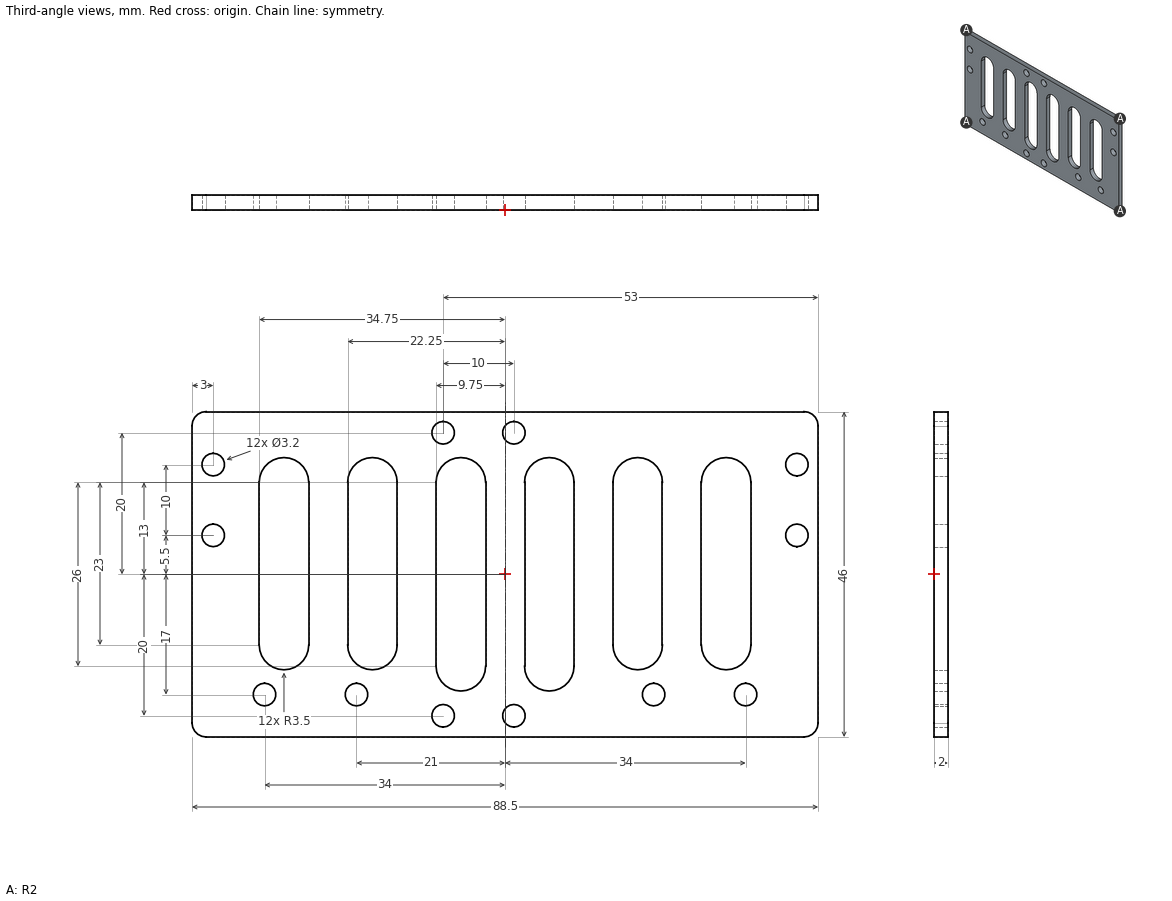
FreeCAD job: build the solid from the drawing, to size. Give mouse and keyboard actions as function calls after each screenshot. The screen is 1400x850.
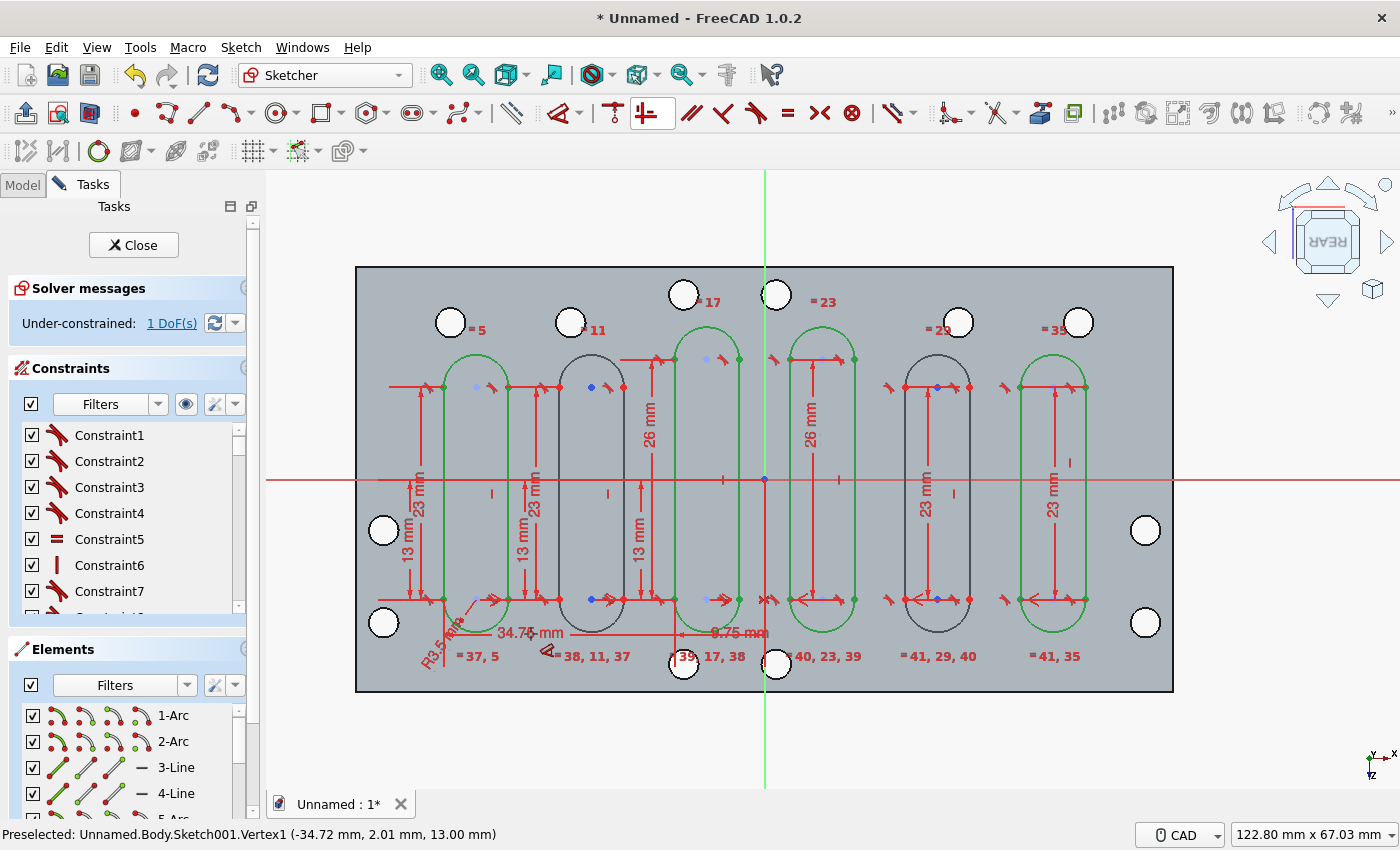
click(559, 600)
click(662, 634)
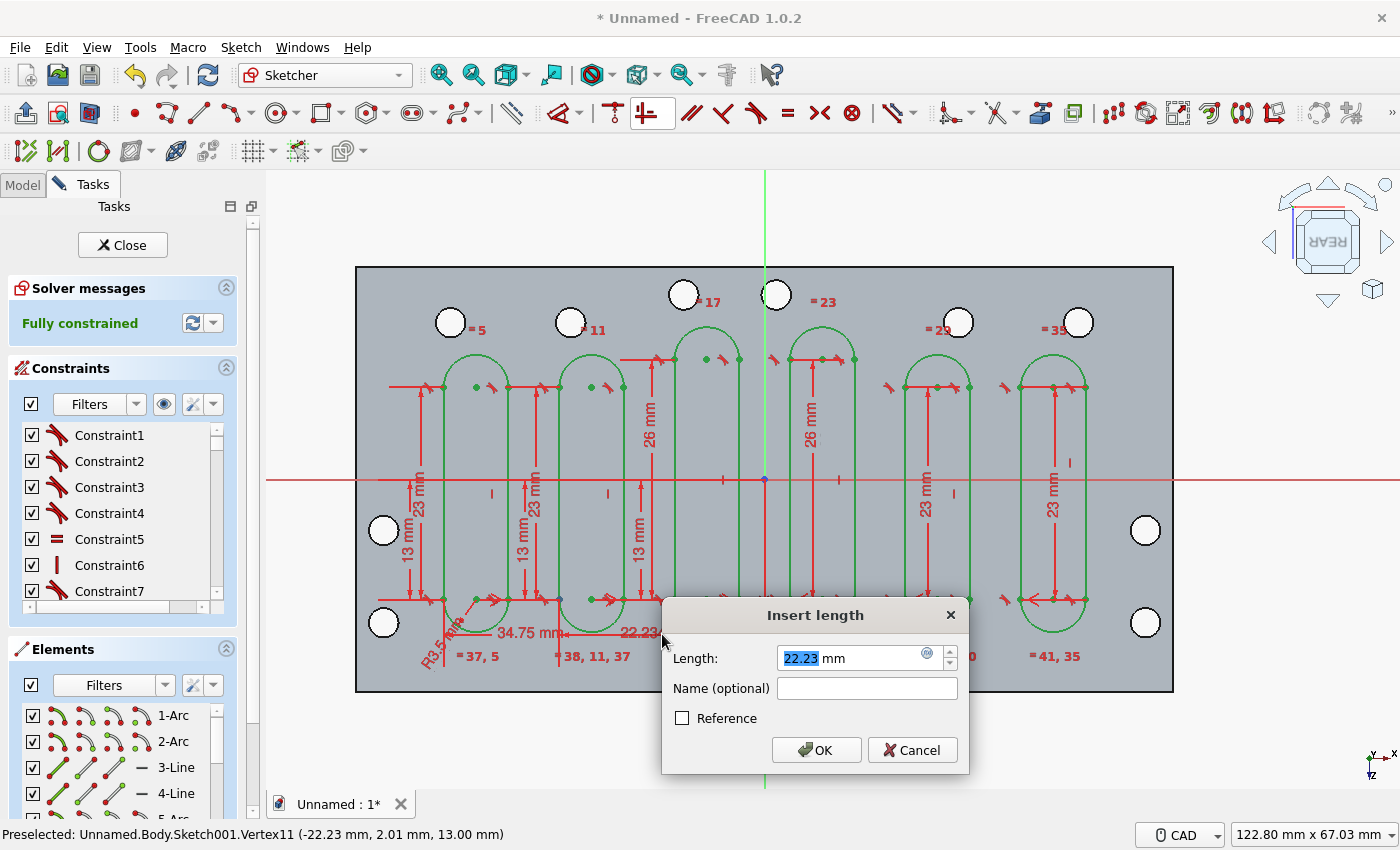
text(22.25)
key(Return)
key(Escape)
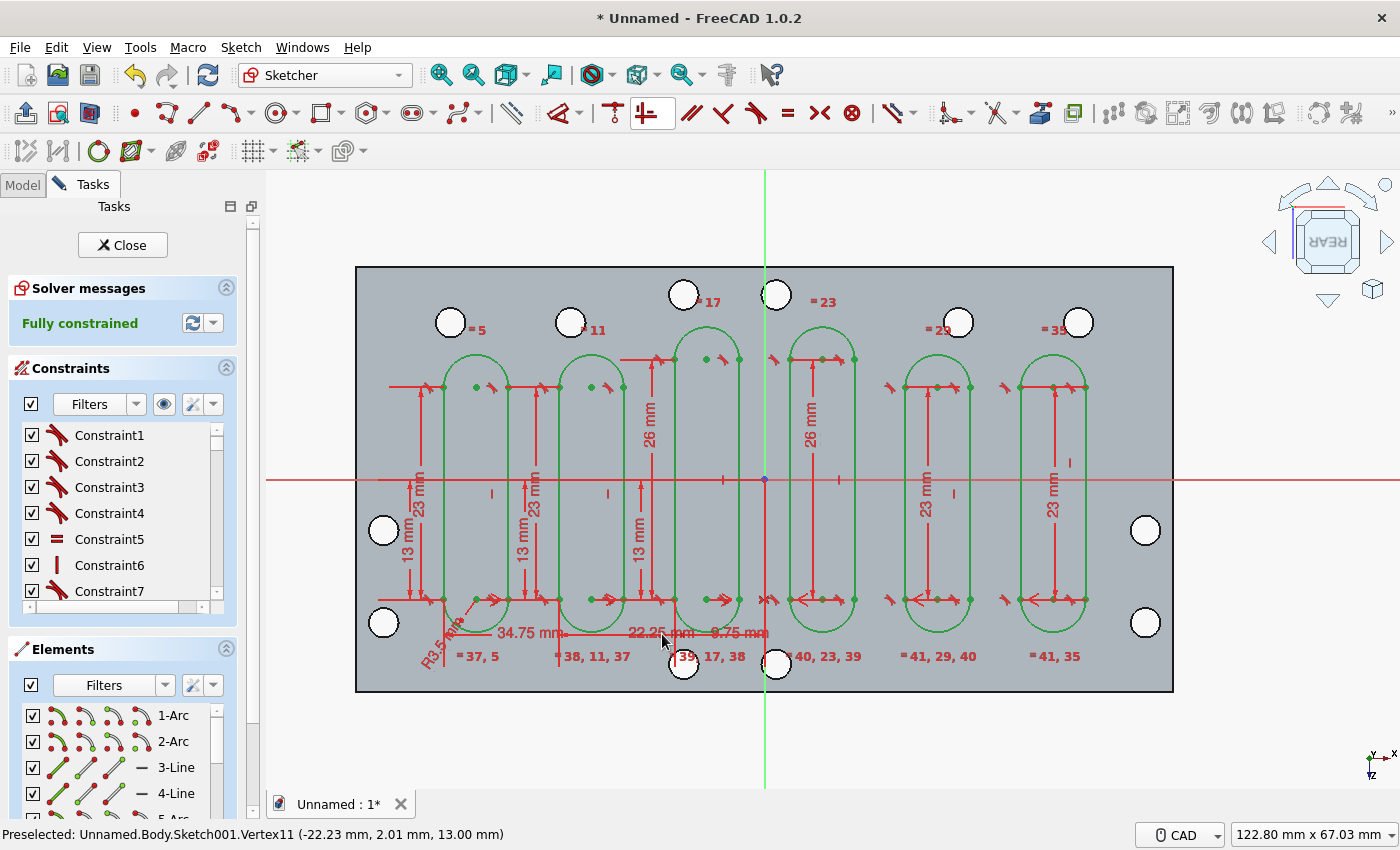
click(123, 245)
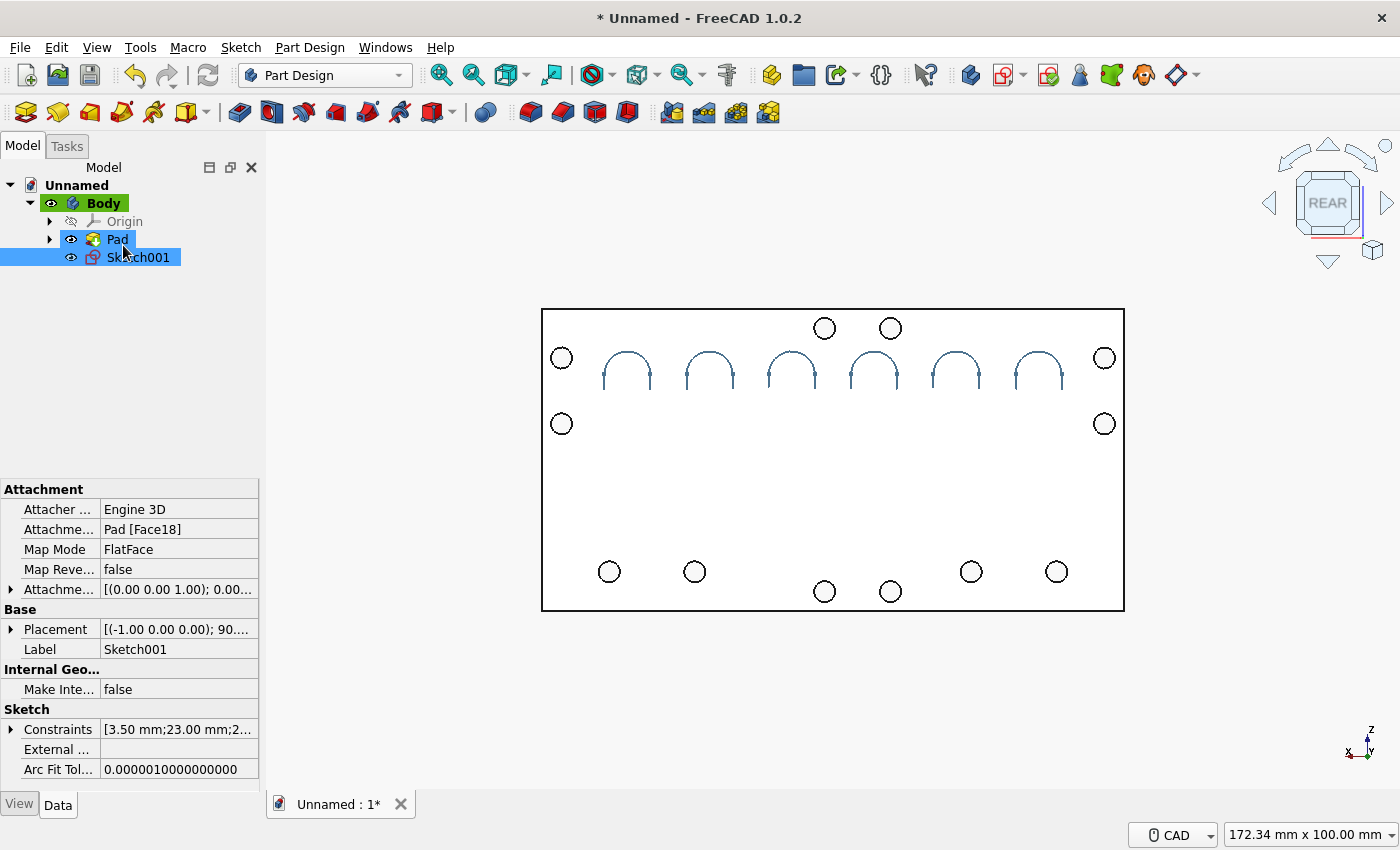
click(240, 112)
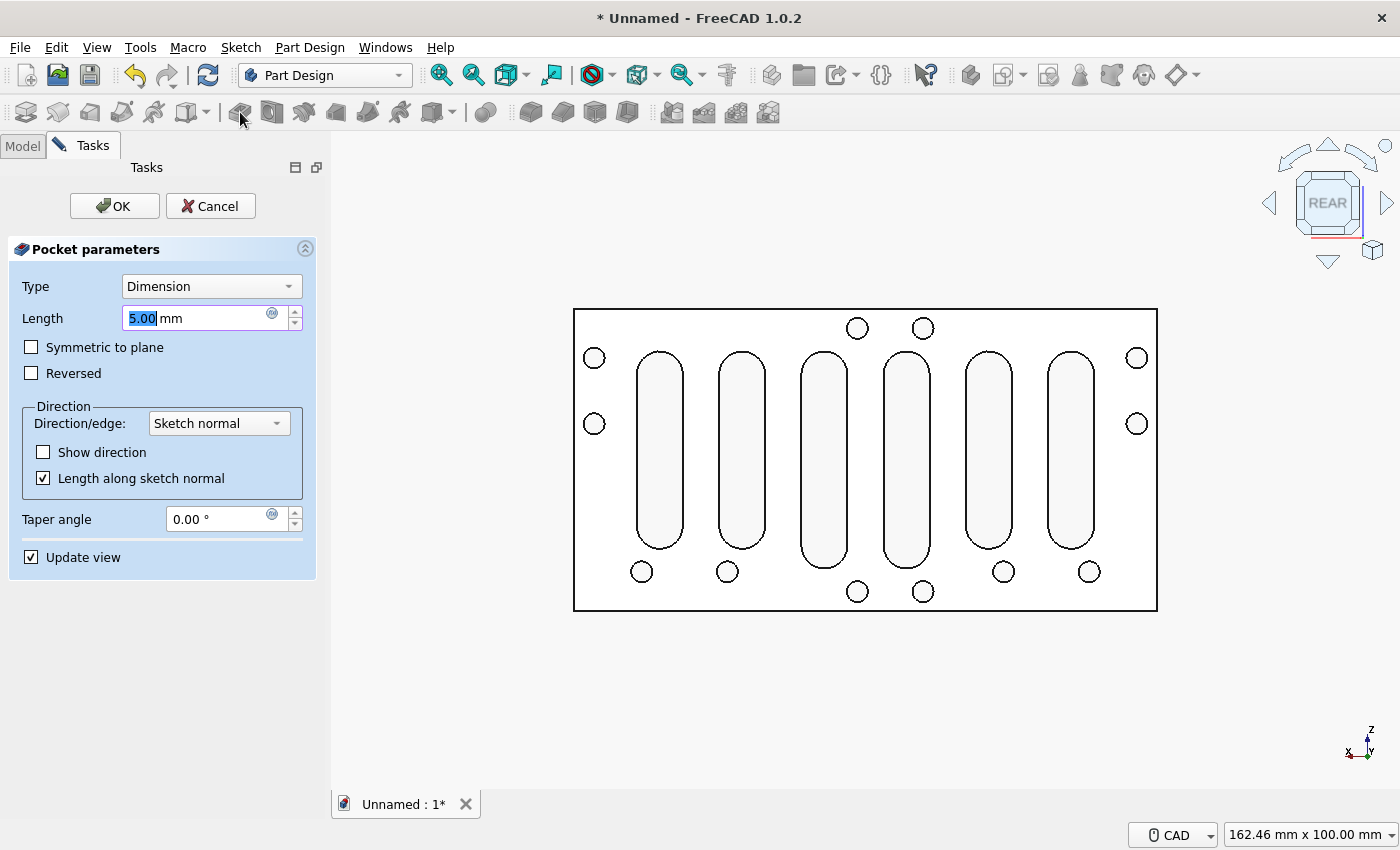
click(212, 286)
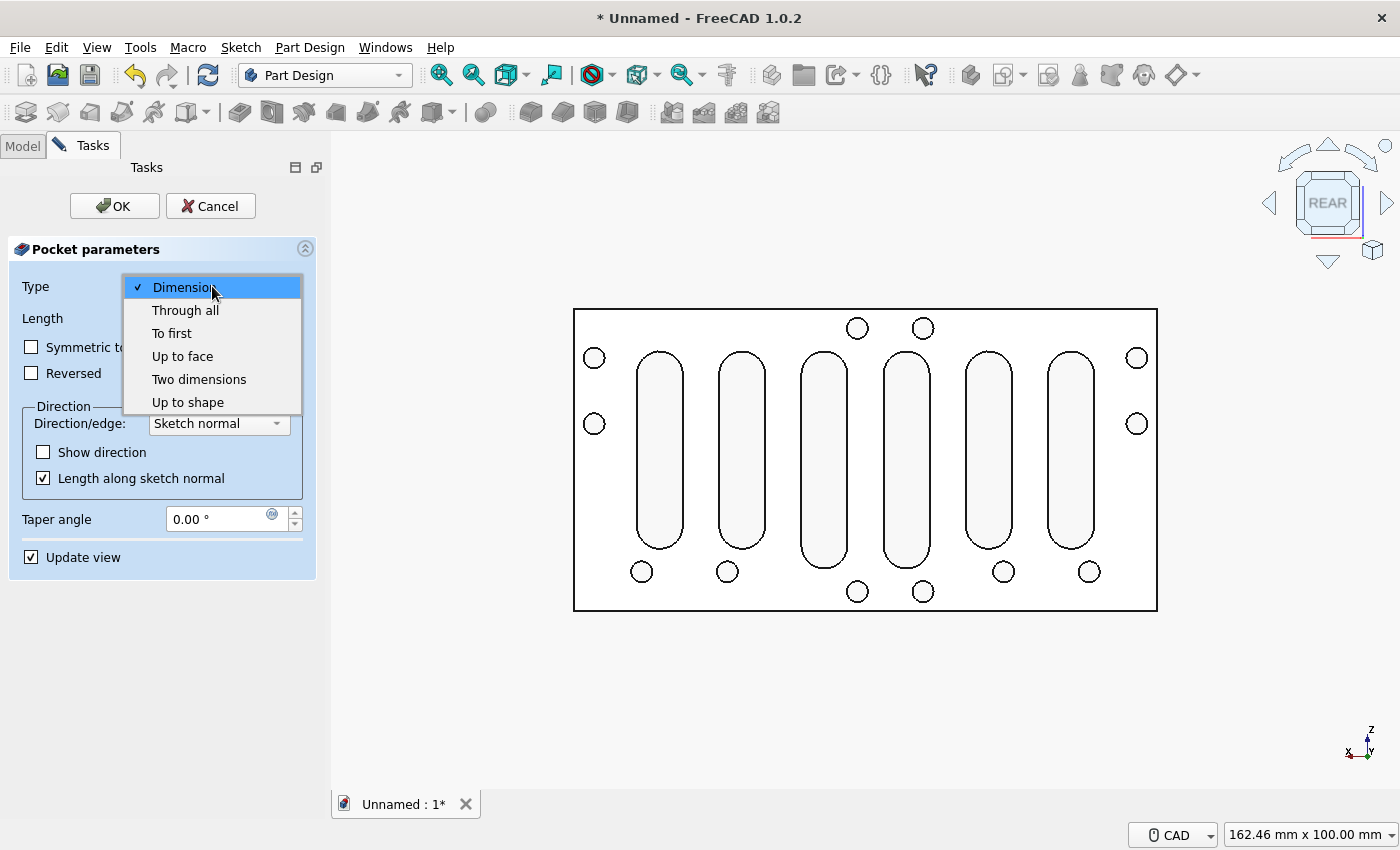
click(212, 310)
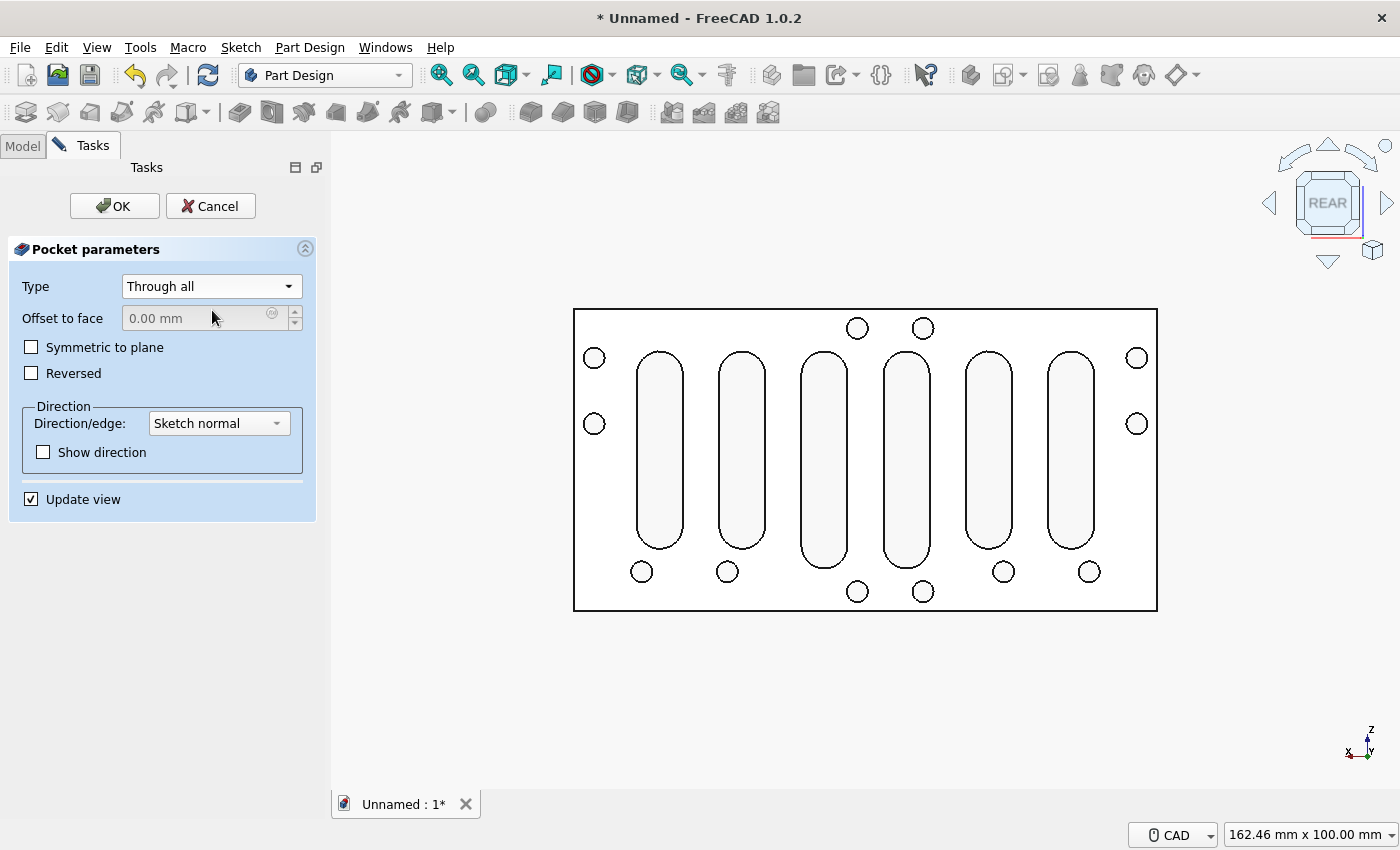
click(115, 206)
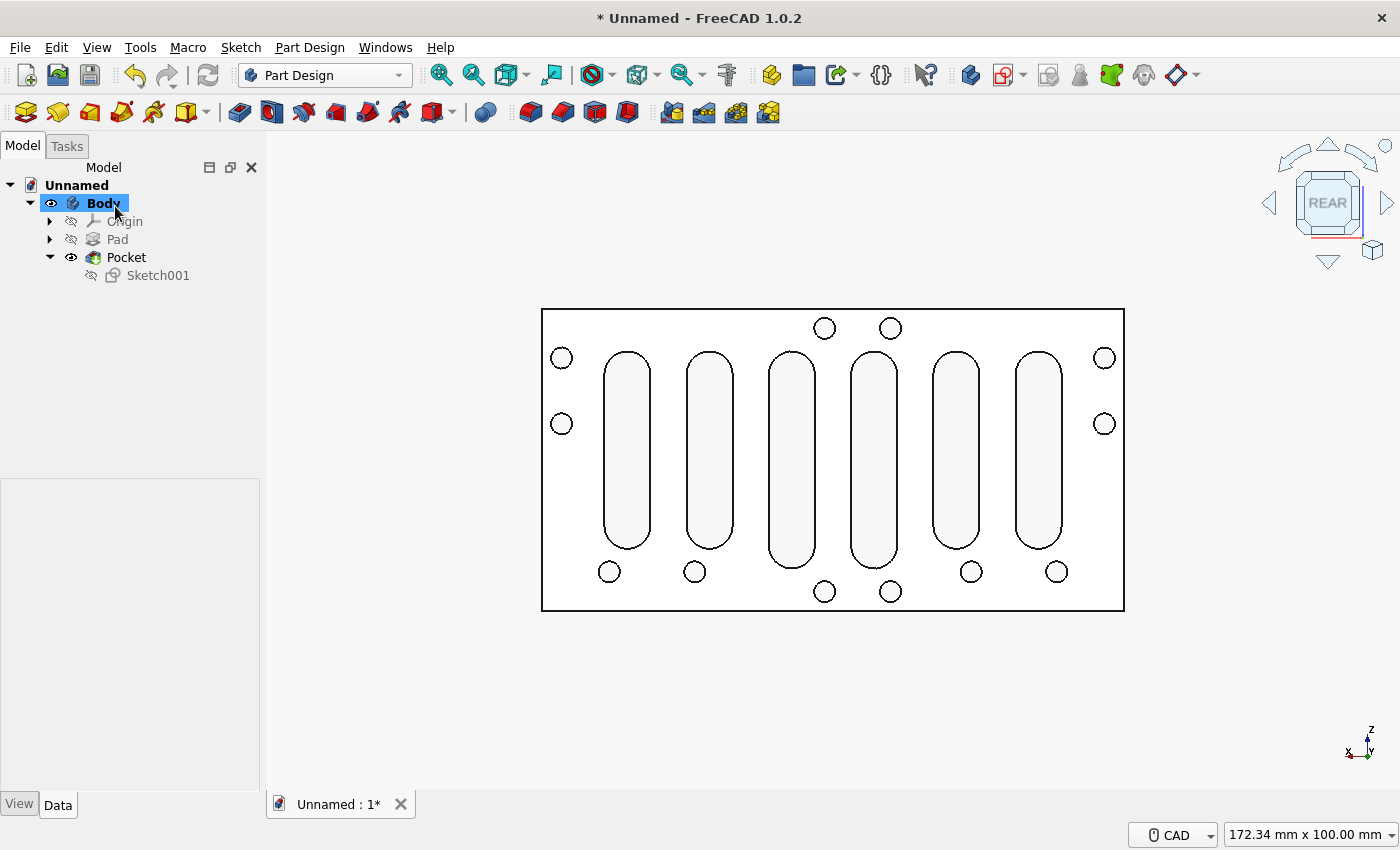
scroll(542, 308, up, 6)